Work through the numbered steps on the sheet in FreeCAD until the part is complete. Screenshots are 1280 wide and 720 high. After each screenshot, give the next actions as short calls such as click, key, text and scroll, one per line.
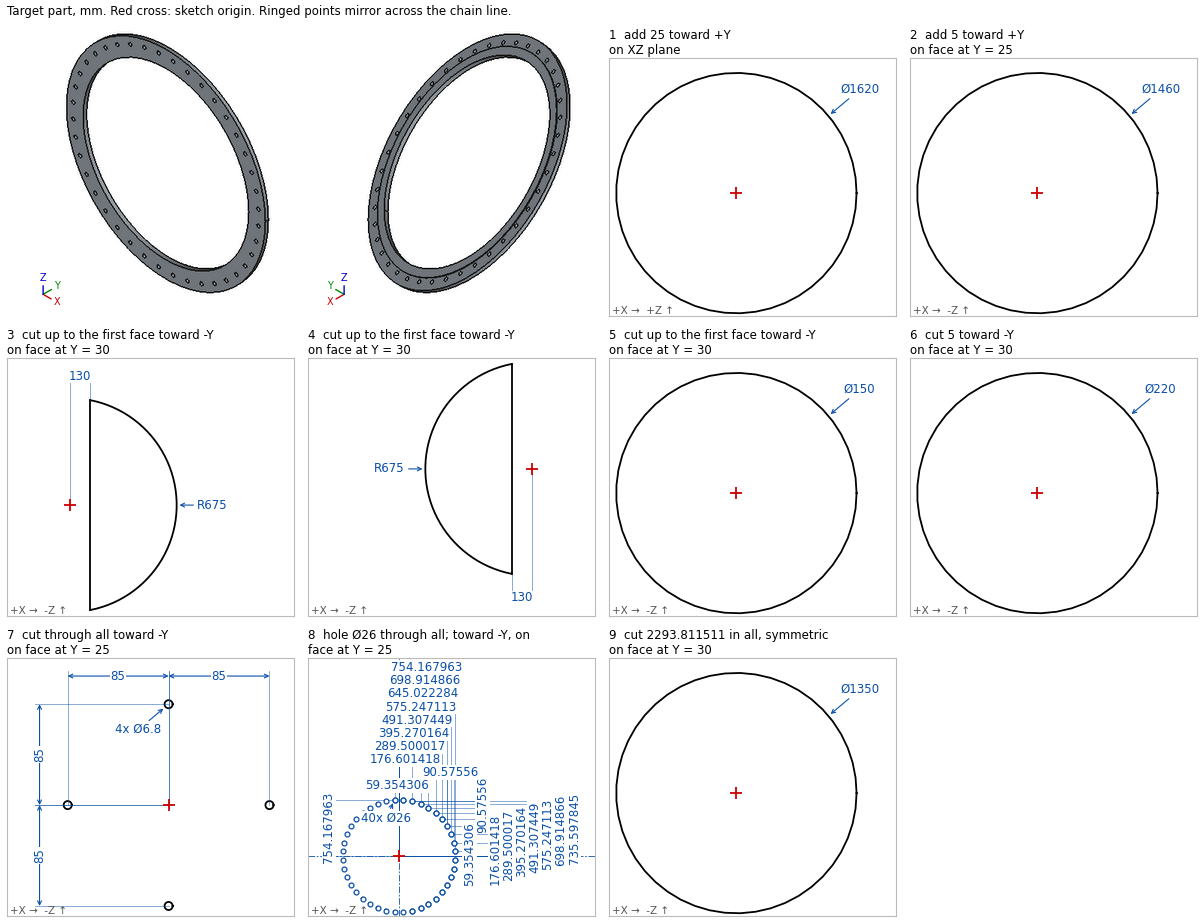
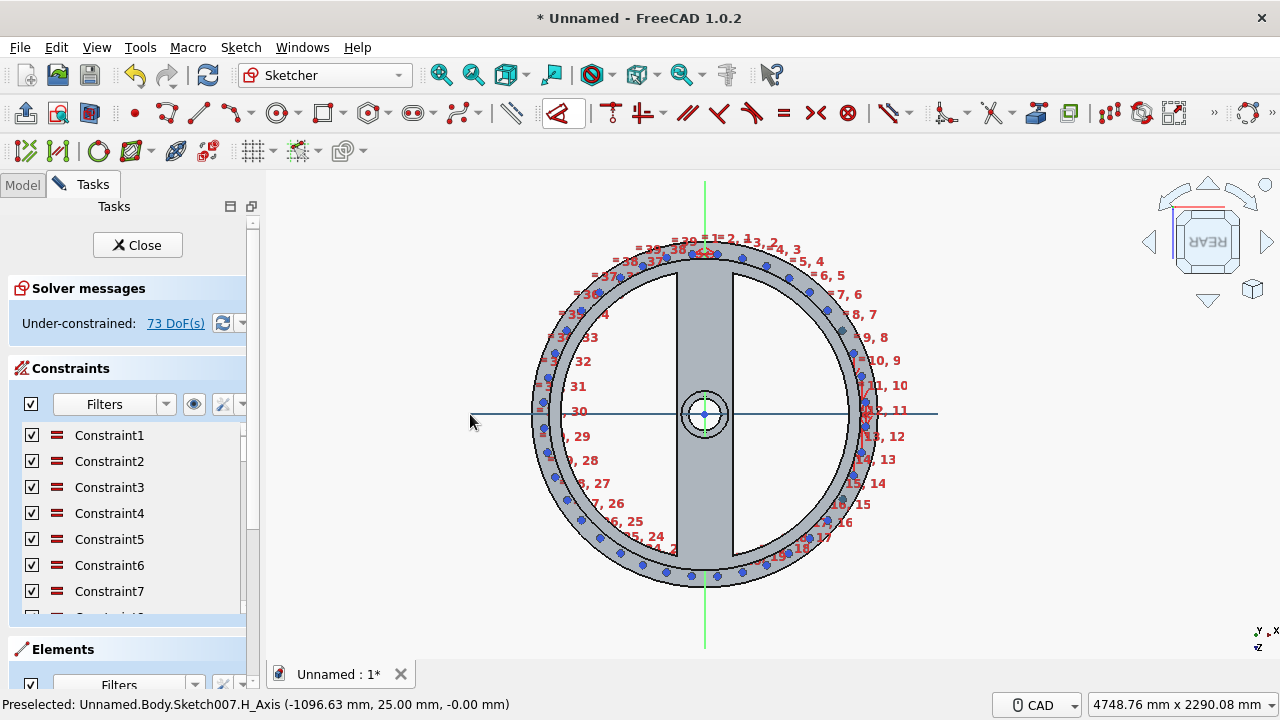
click(816, 114)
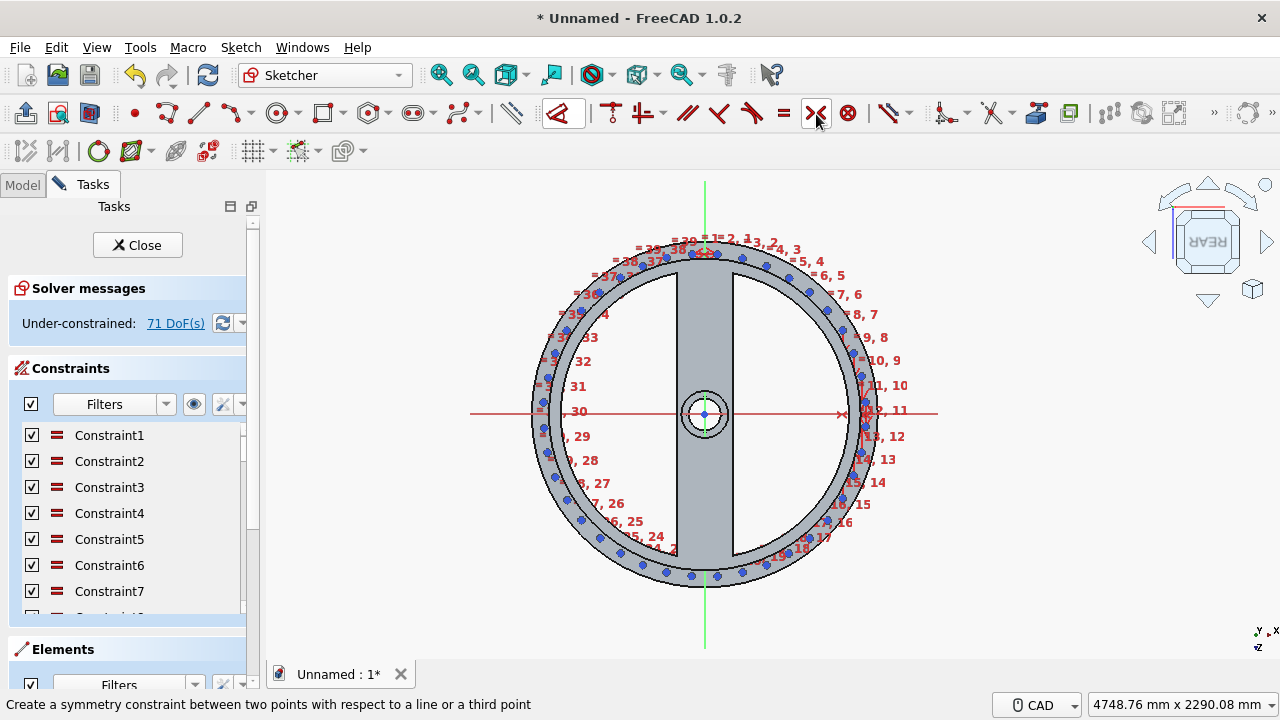
click(828, 311)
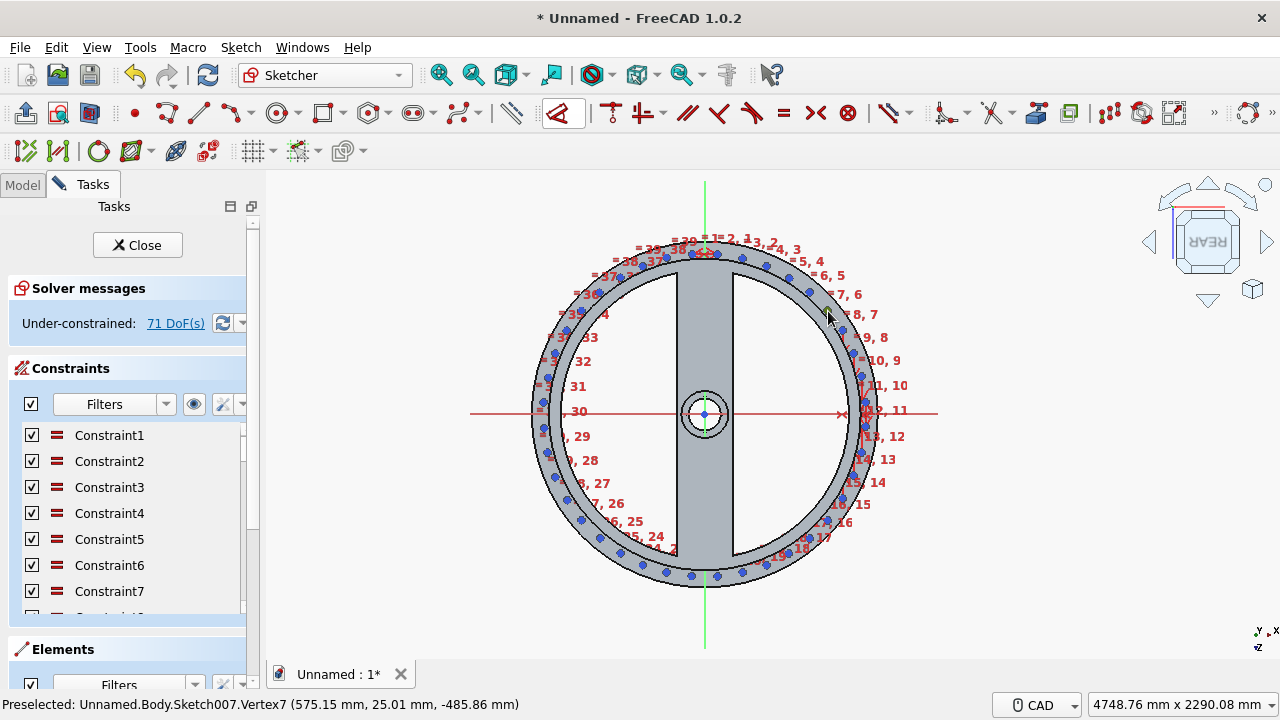
click(828, 521)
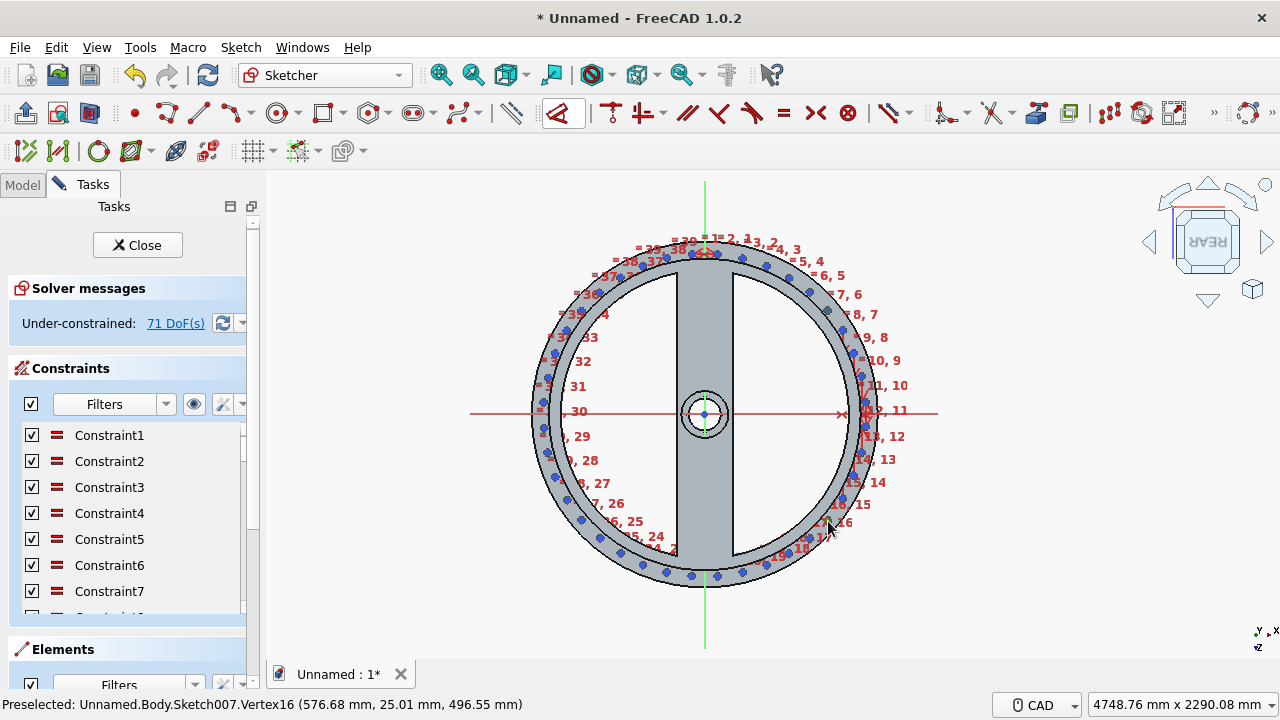
click(470, 414)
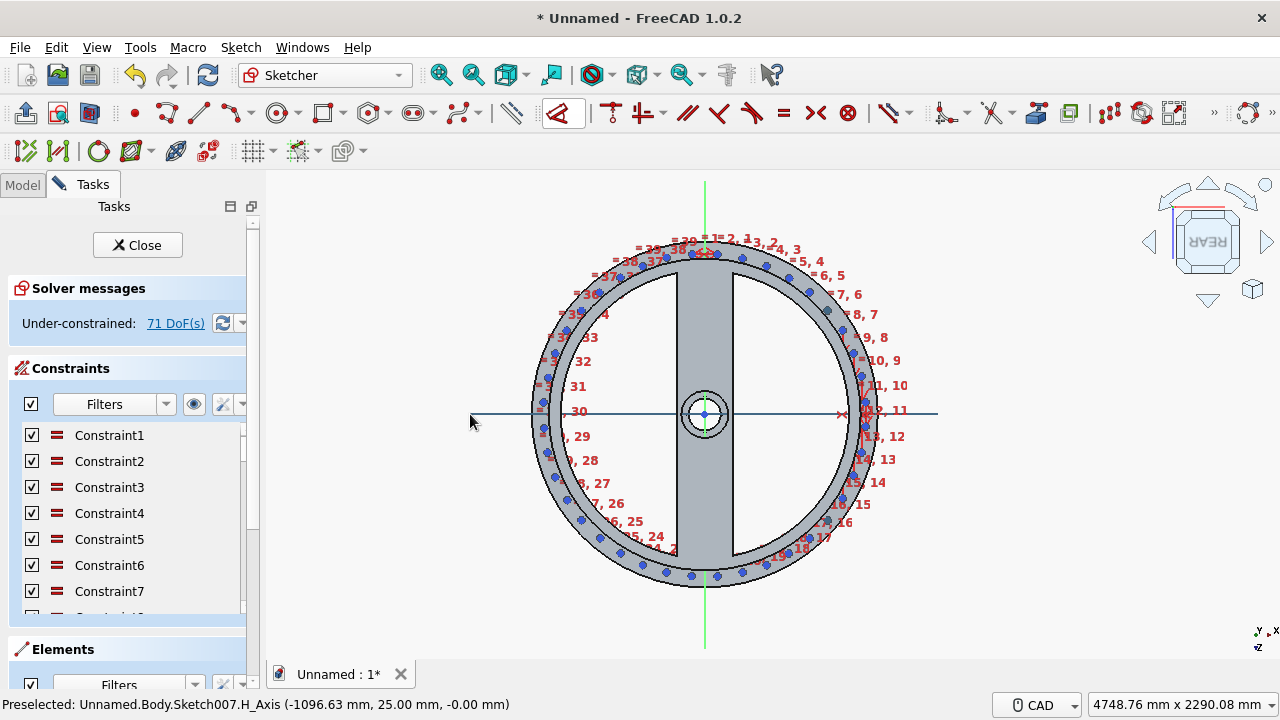
click(816, 114)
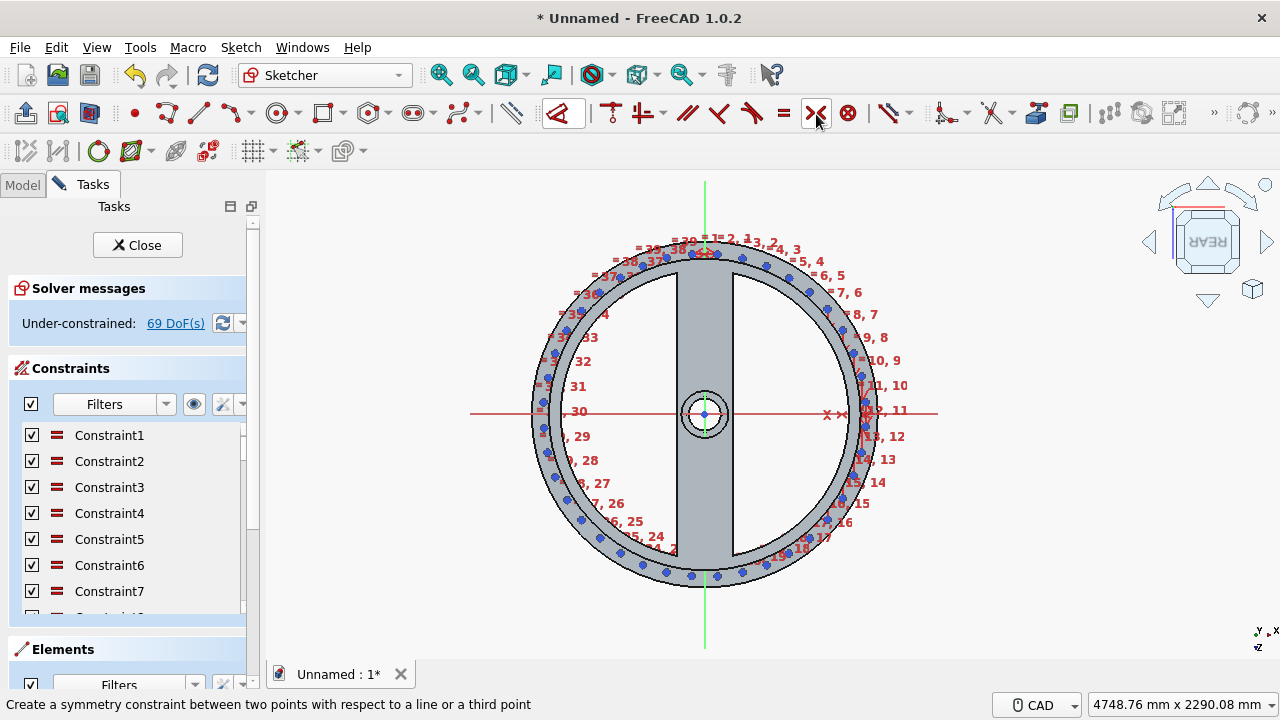
click(810, 292)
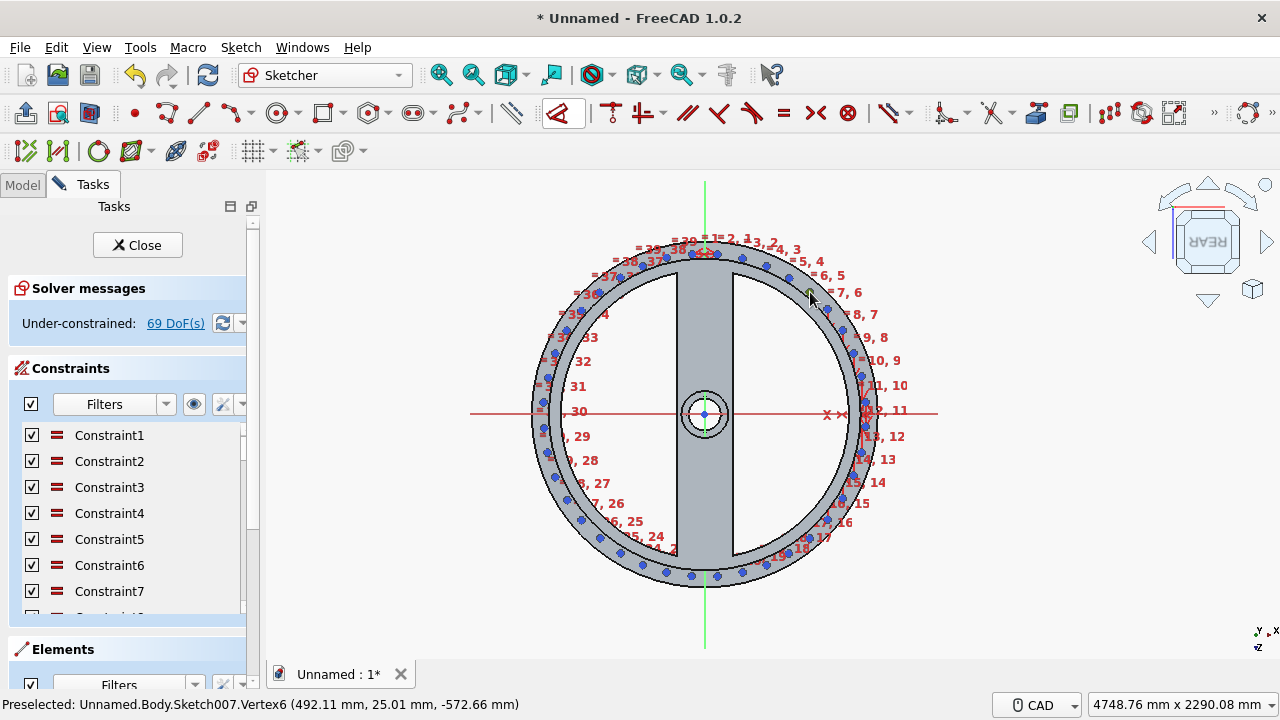
click(810, 539)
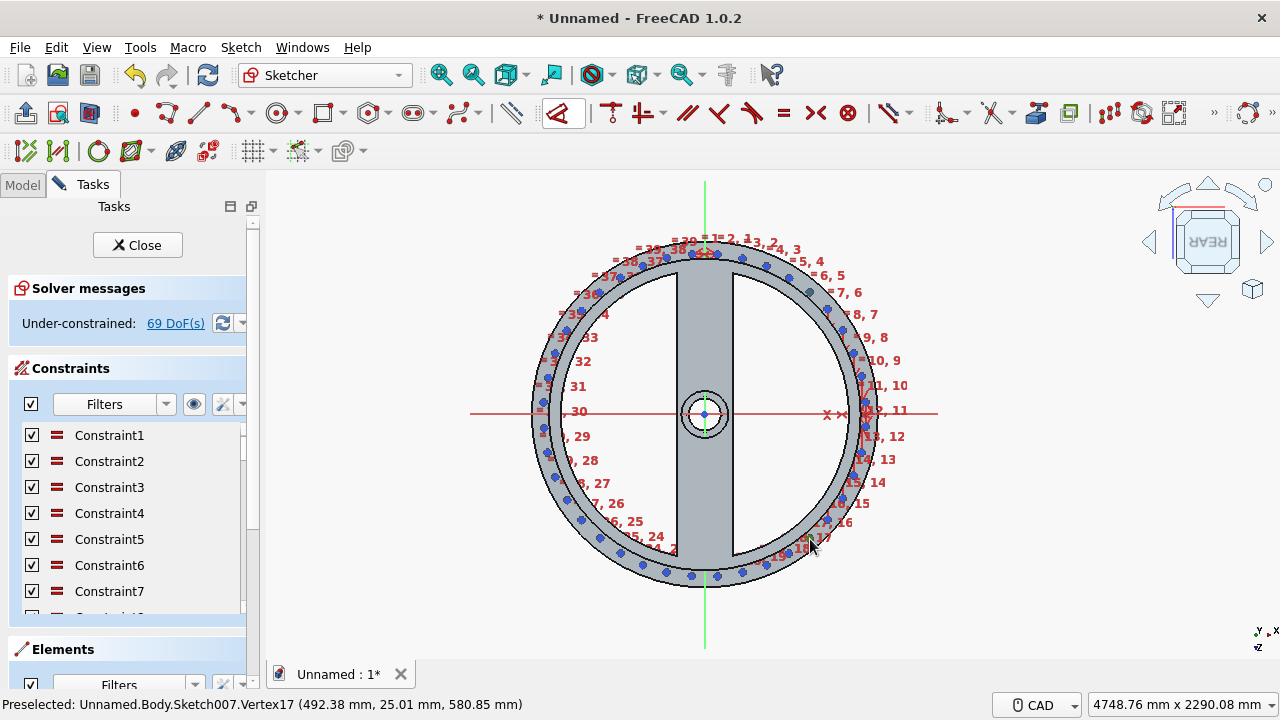
click(470, 414)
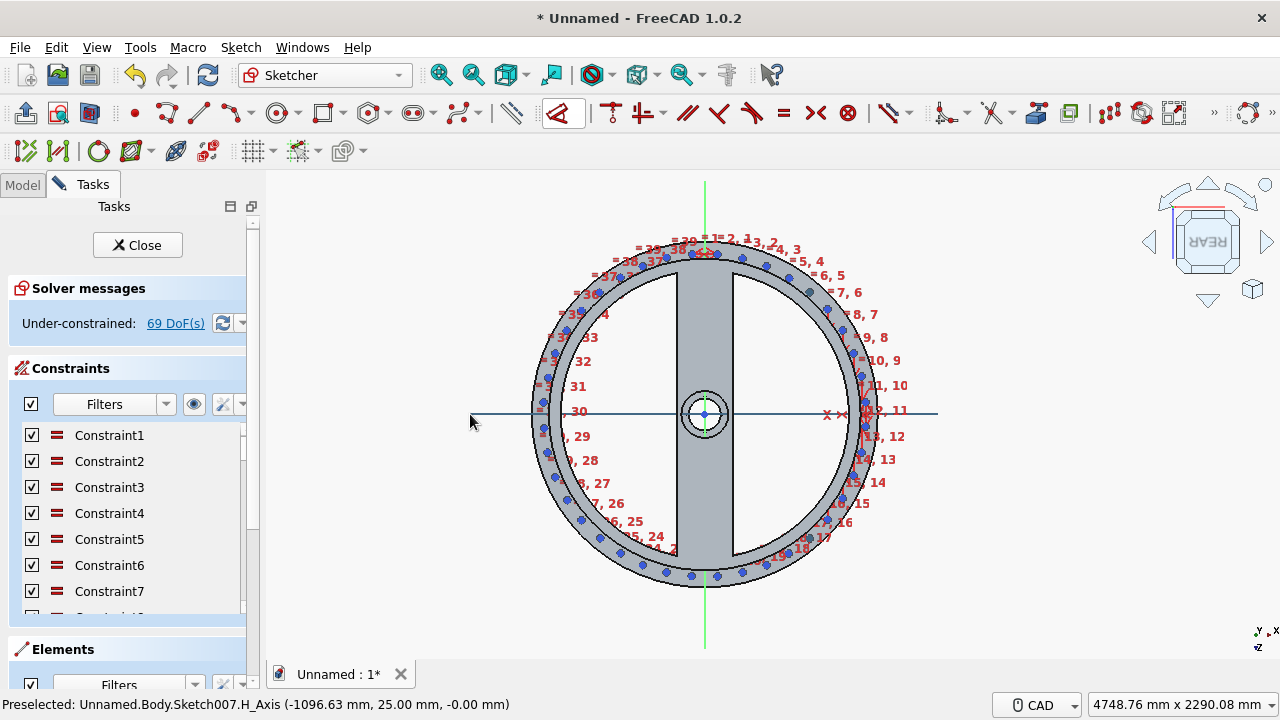
key(s)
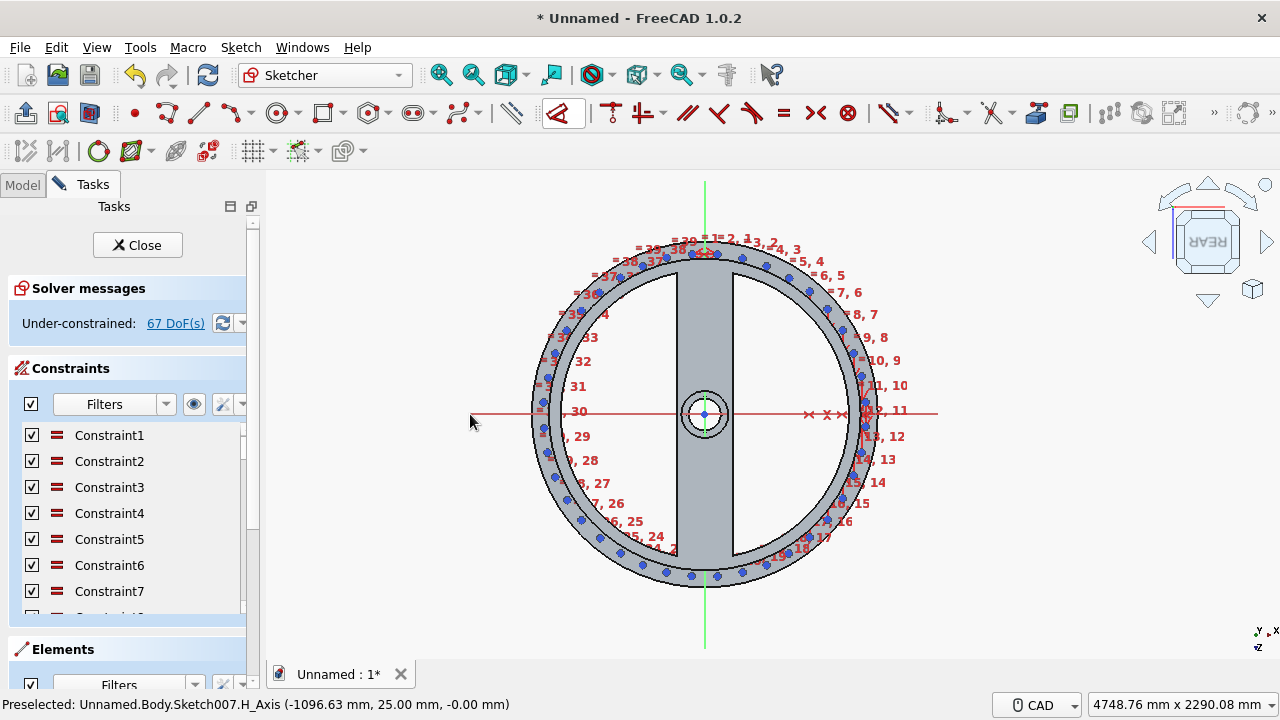
click(789, 278)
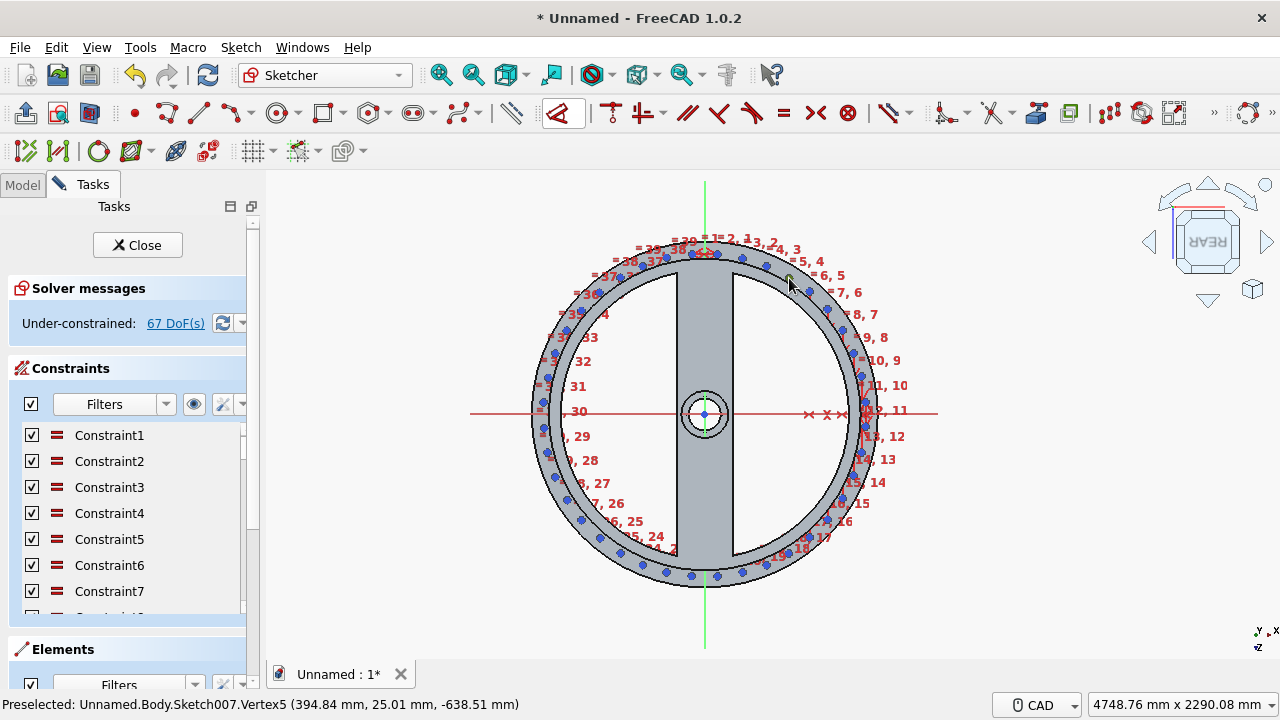
click(789, 554)